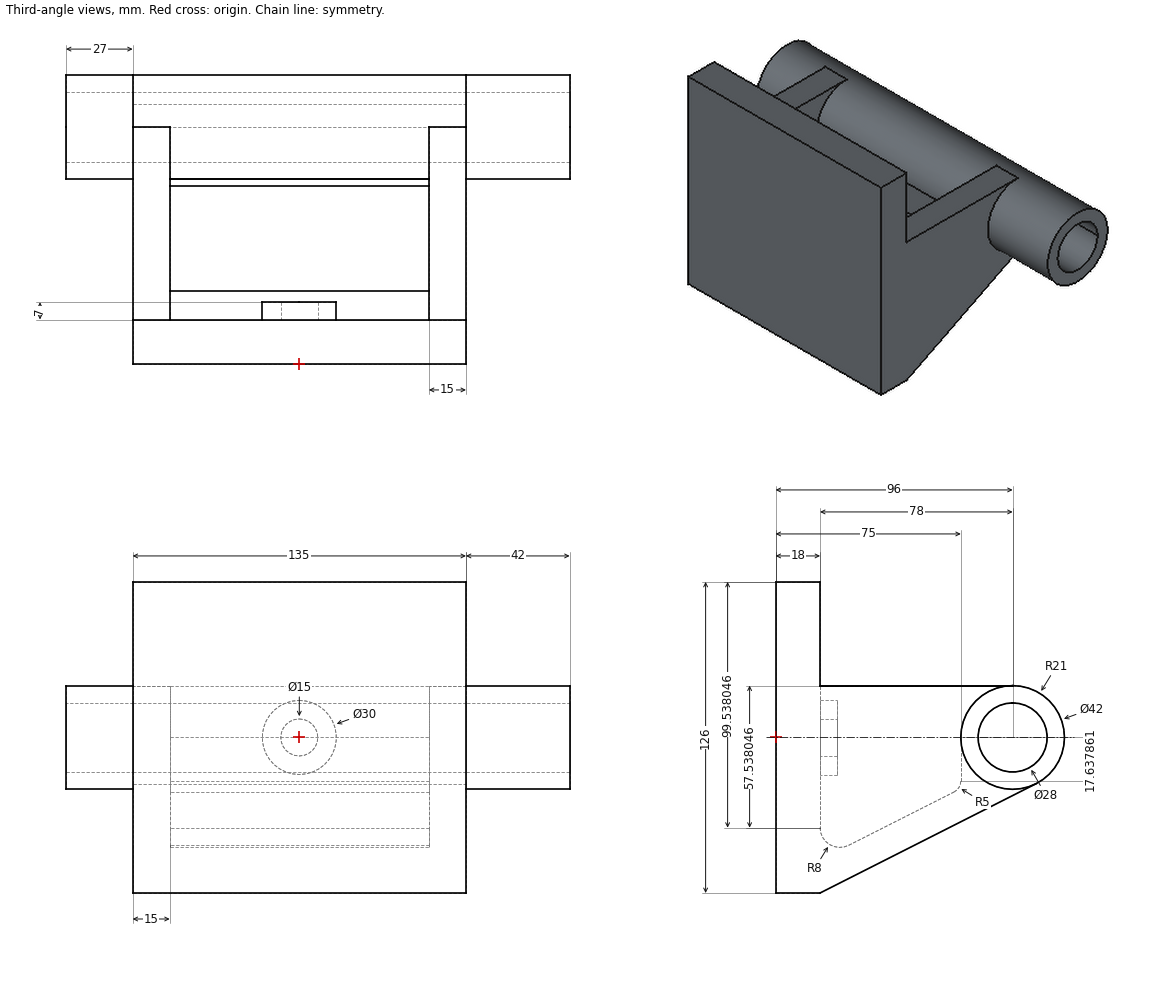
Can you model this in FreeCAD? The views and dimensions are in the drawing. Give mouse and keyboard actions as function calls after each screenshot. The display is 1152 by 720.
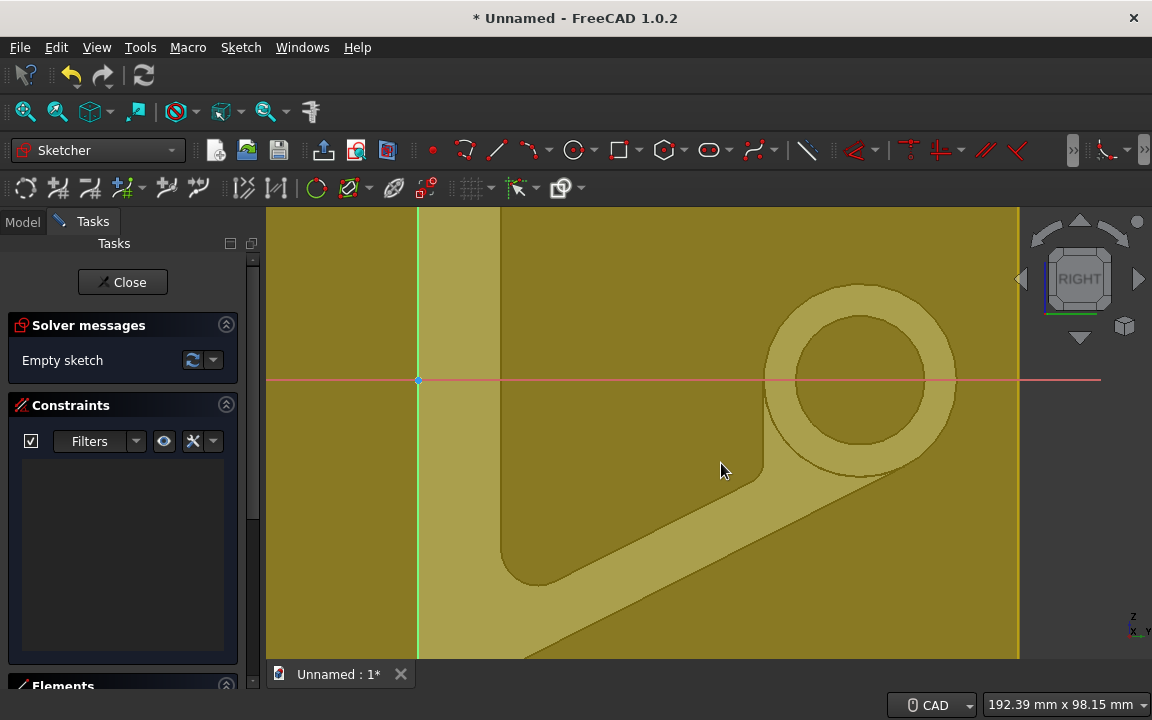
click(498, 150)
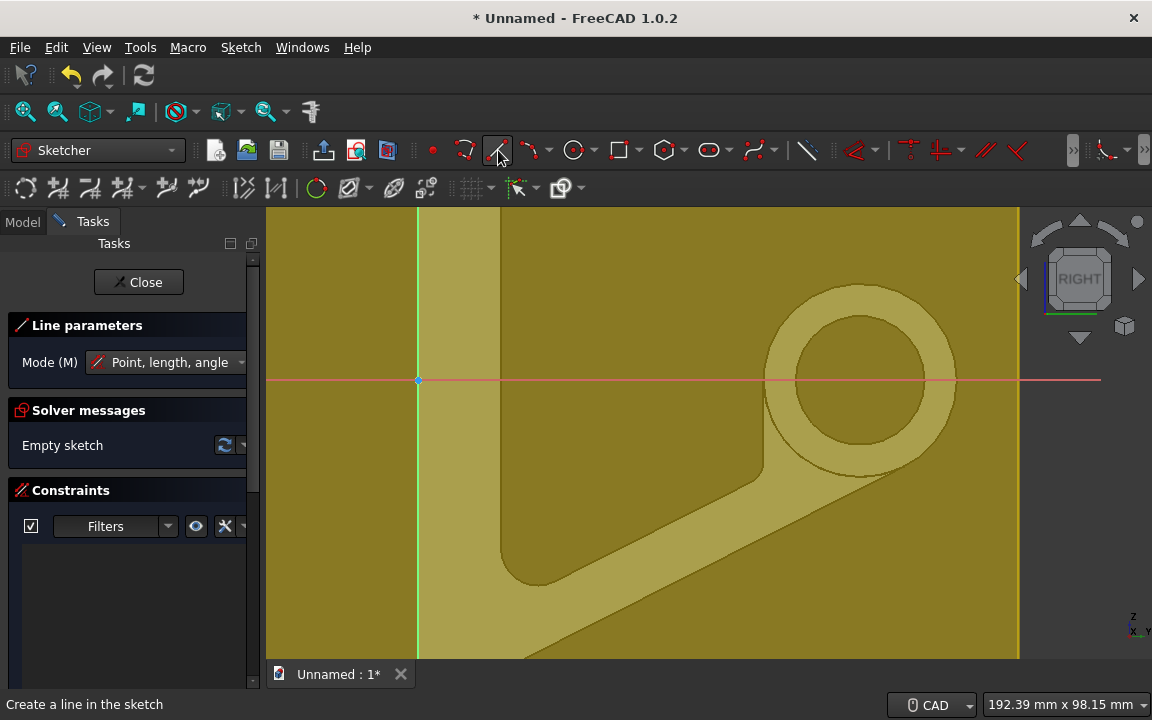
click(763, 380)
click(763, 462)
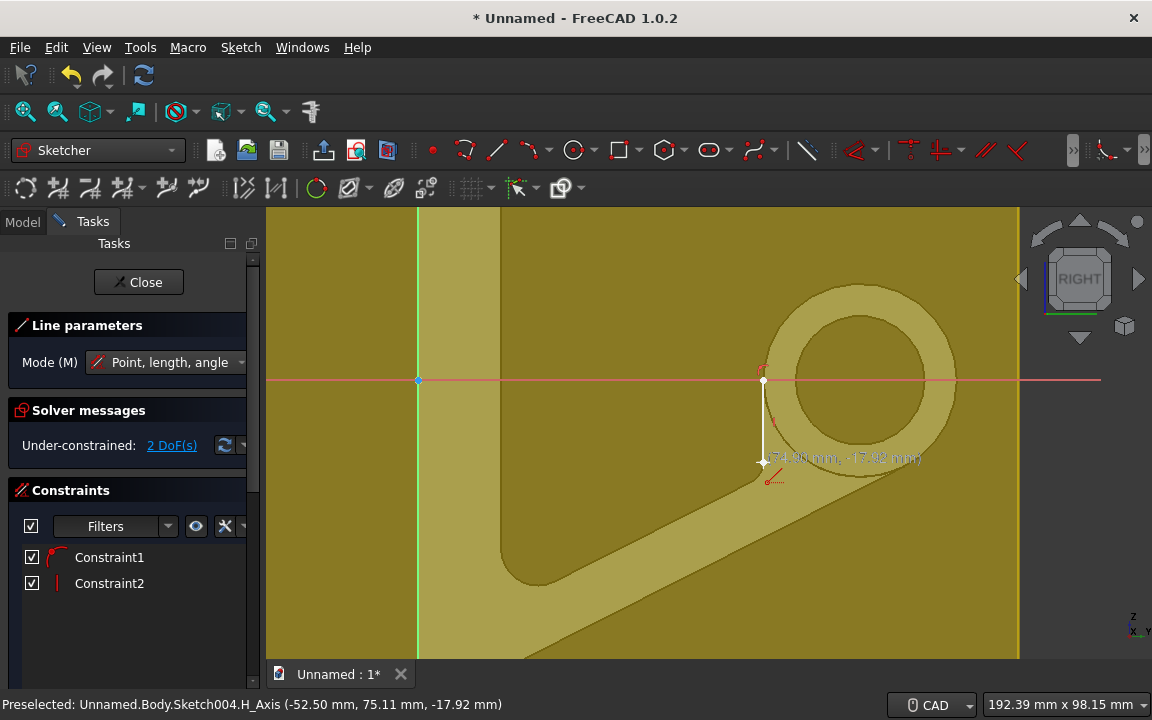
click(751, 482)
click(554, 582)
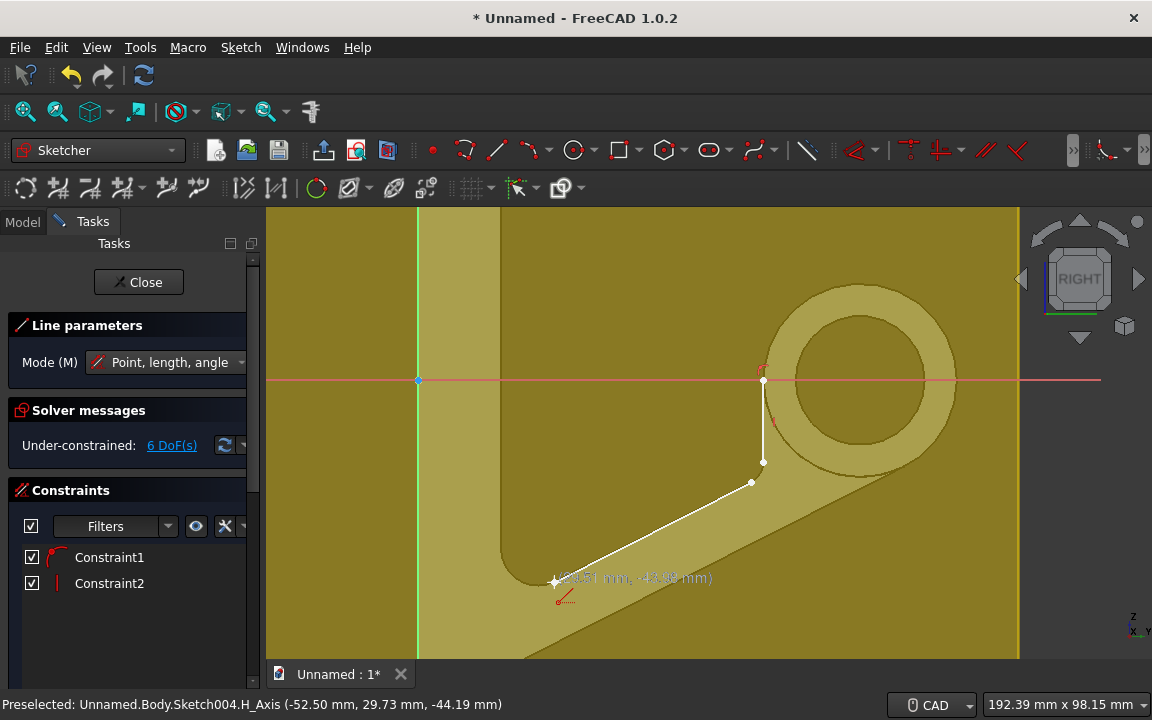
click(466, 150)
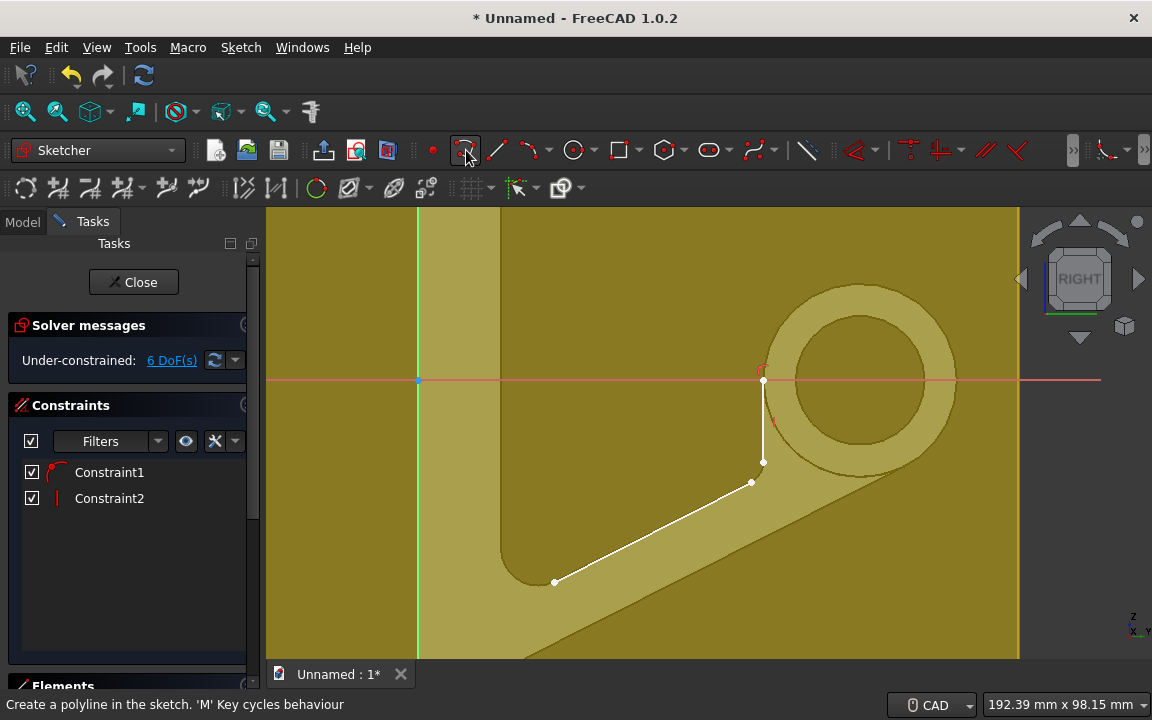
click(501, 549)
click(501, 284)
click(860, 284)
right_click(860, 284)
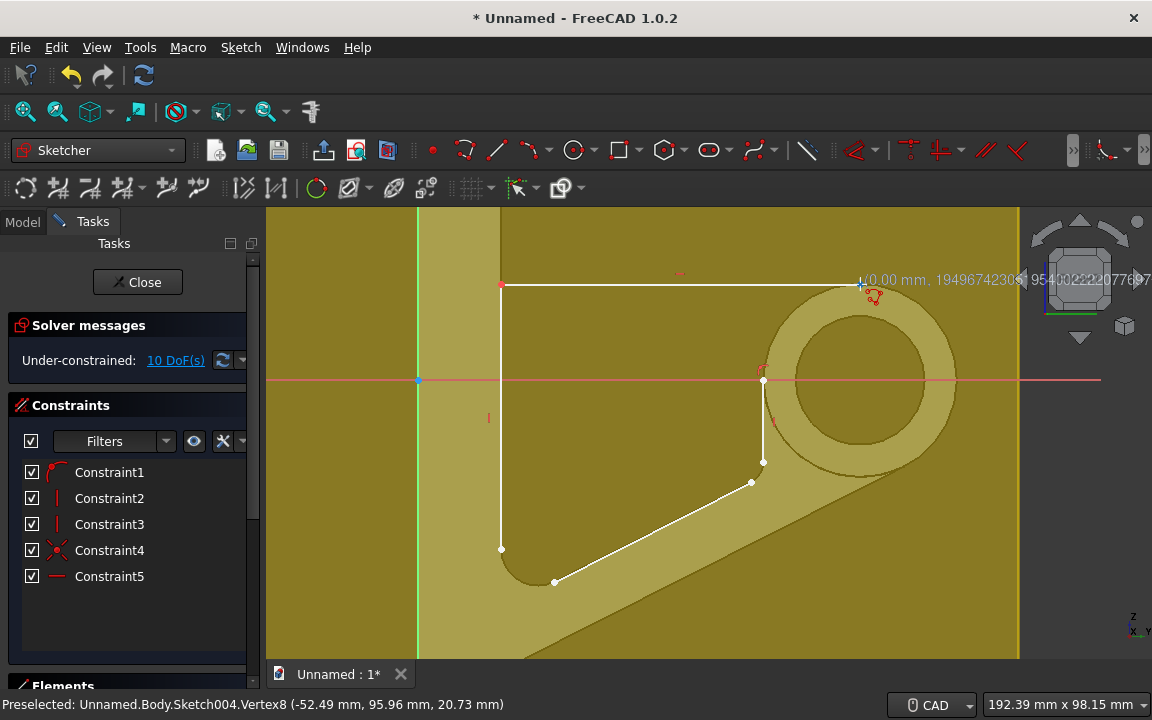
click(530, 150)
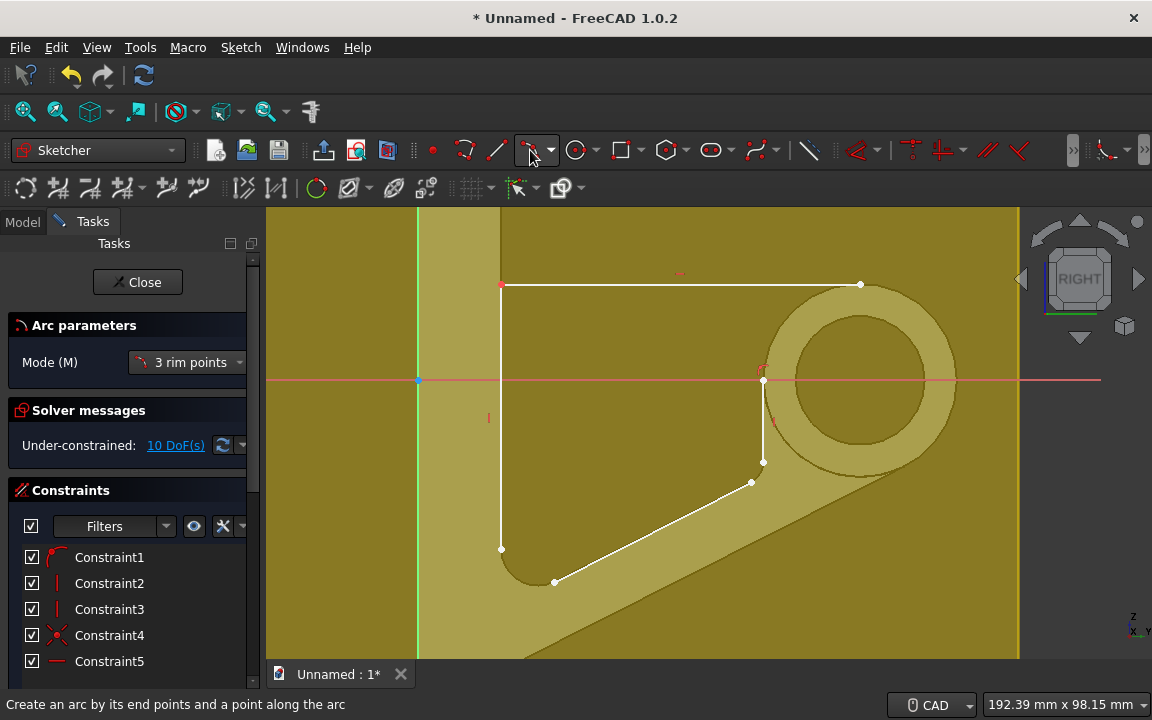
click(763, 463)
click(751, 483)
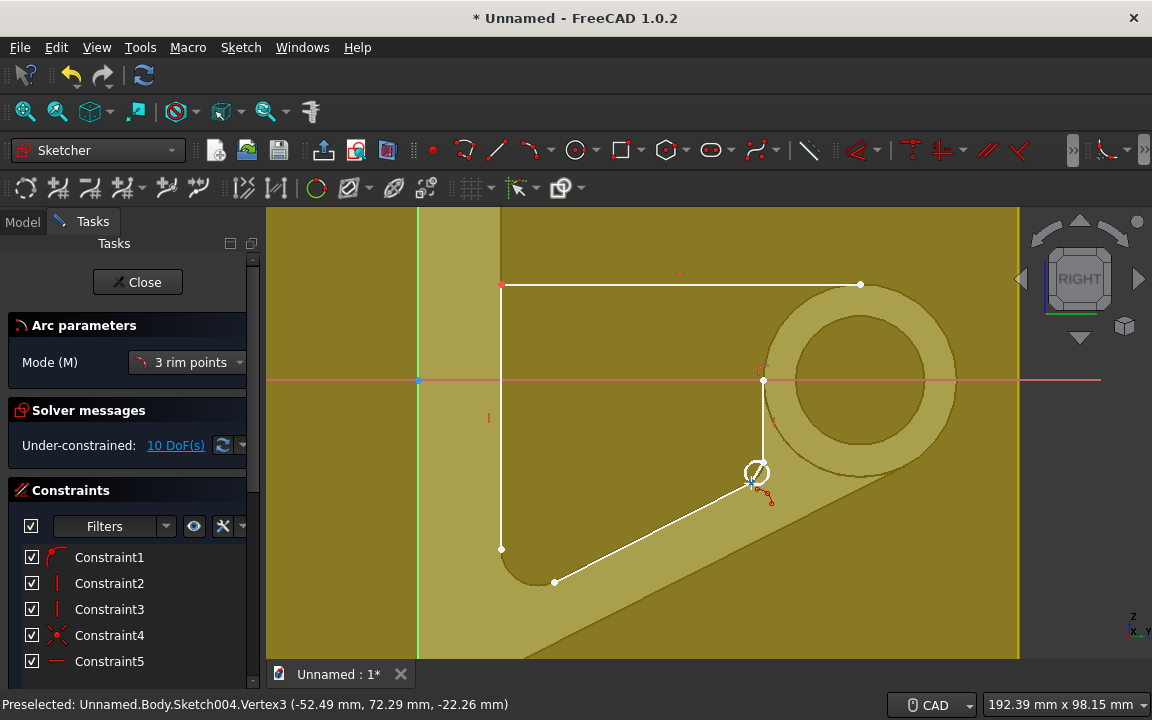
scroll(760, 474, up, 8)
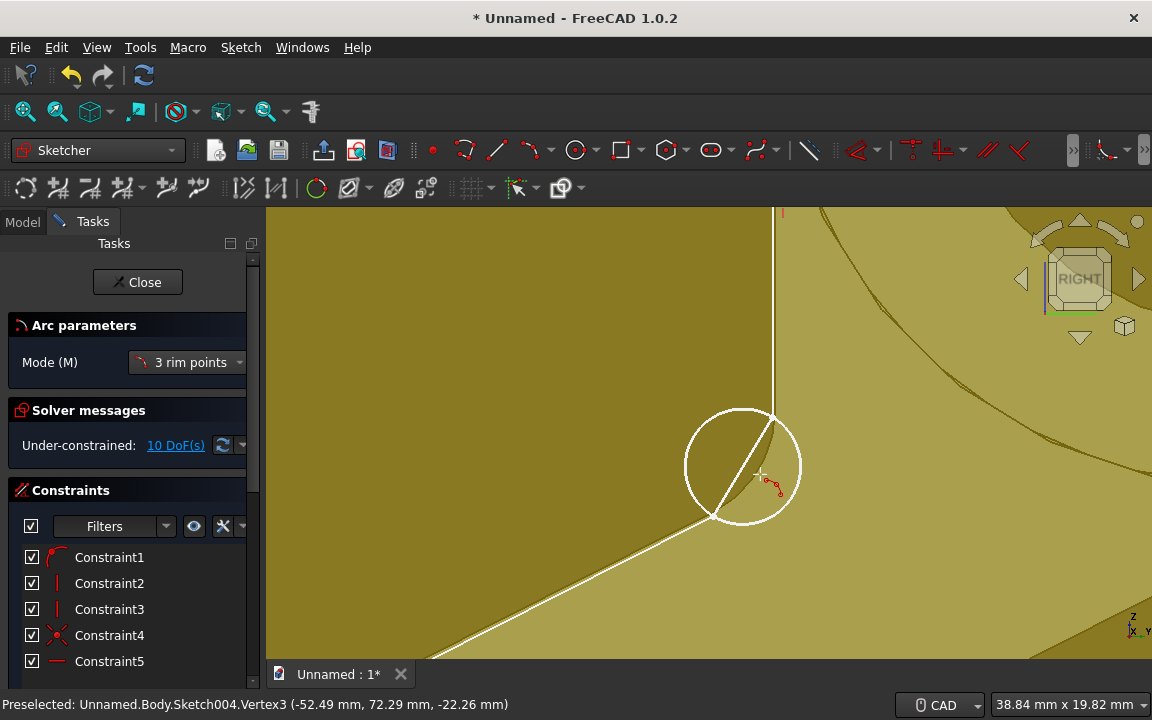
click(758, 470)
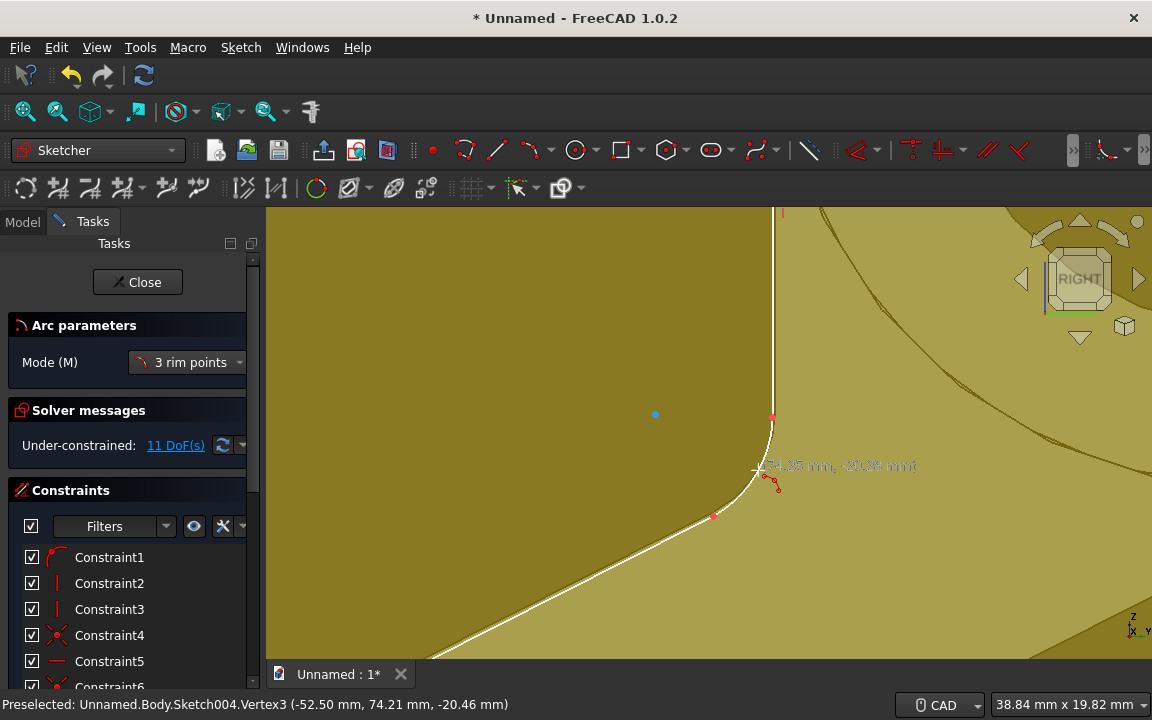
scroll(762, 475, down, 8)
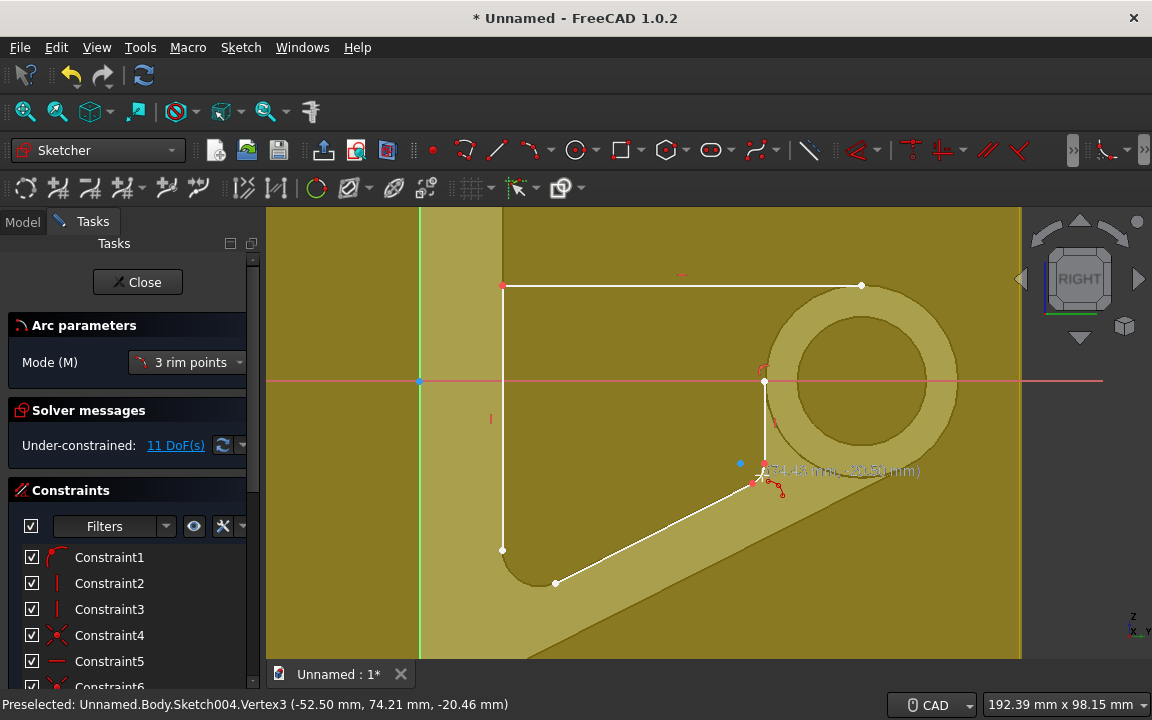
click(556, 584)
click(503, 551)
click(520, 581)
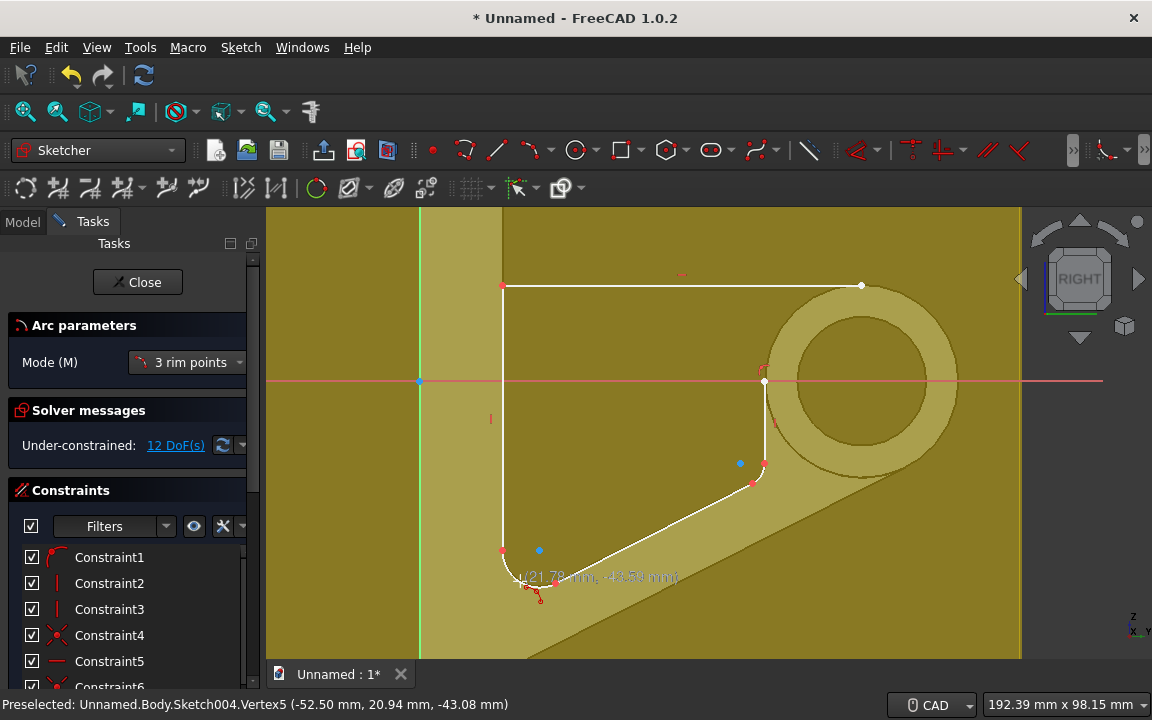
click(862, 286)
click(765, 381)
click(793, 313)
key(Escape)